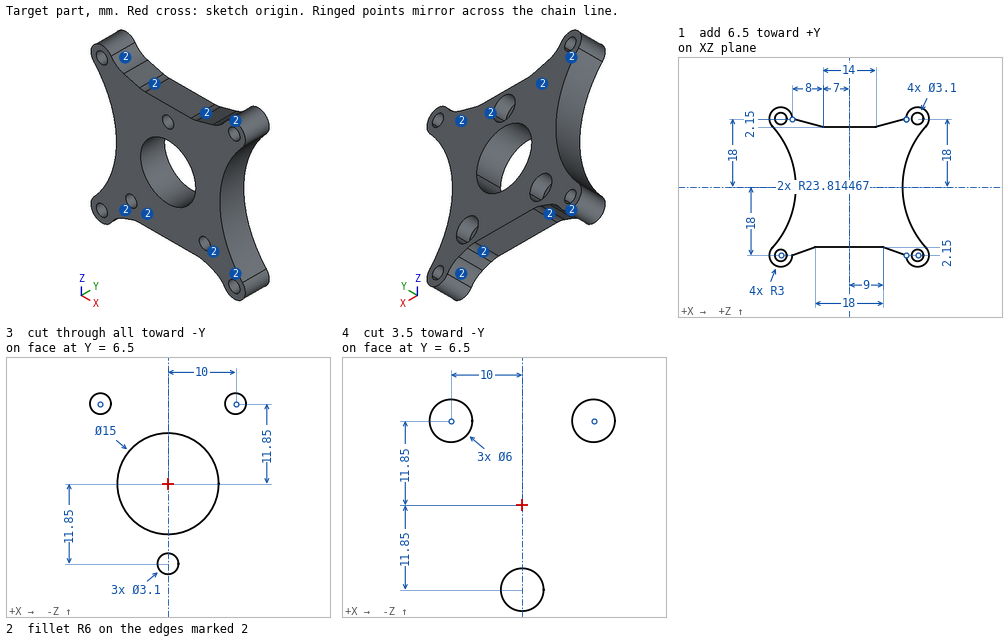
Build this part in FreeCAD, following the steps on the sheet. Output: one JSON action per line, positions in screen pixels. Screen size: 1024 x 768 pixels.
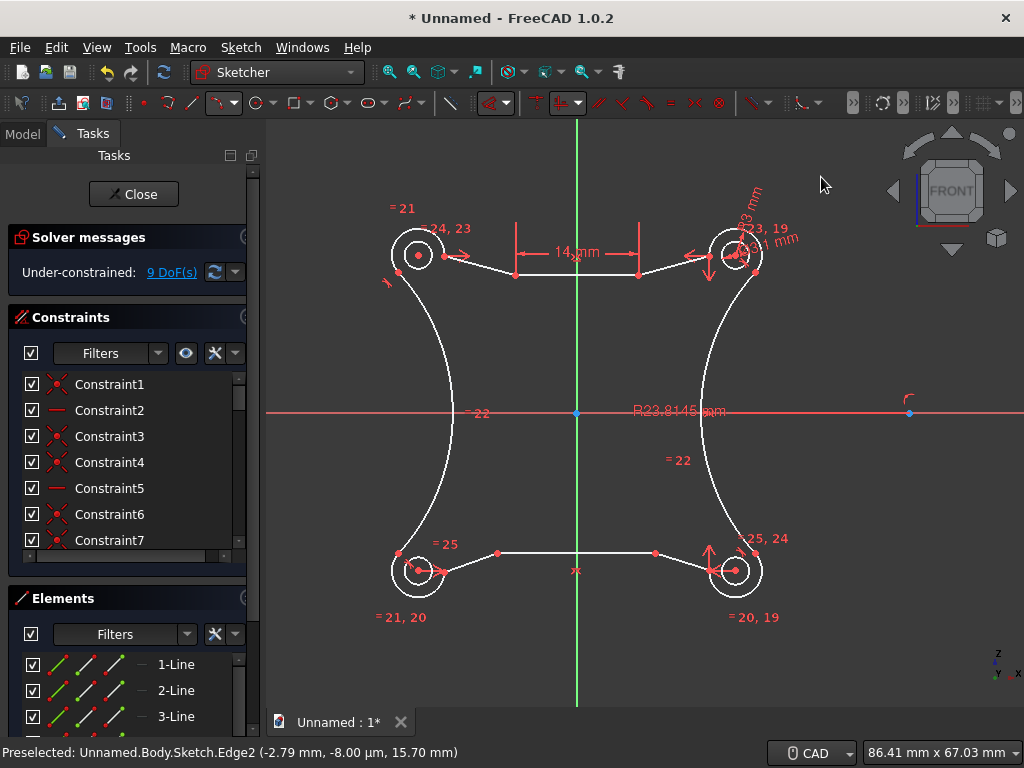
{"action": "left_click", "coordinate": [608, 553]}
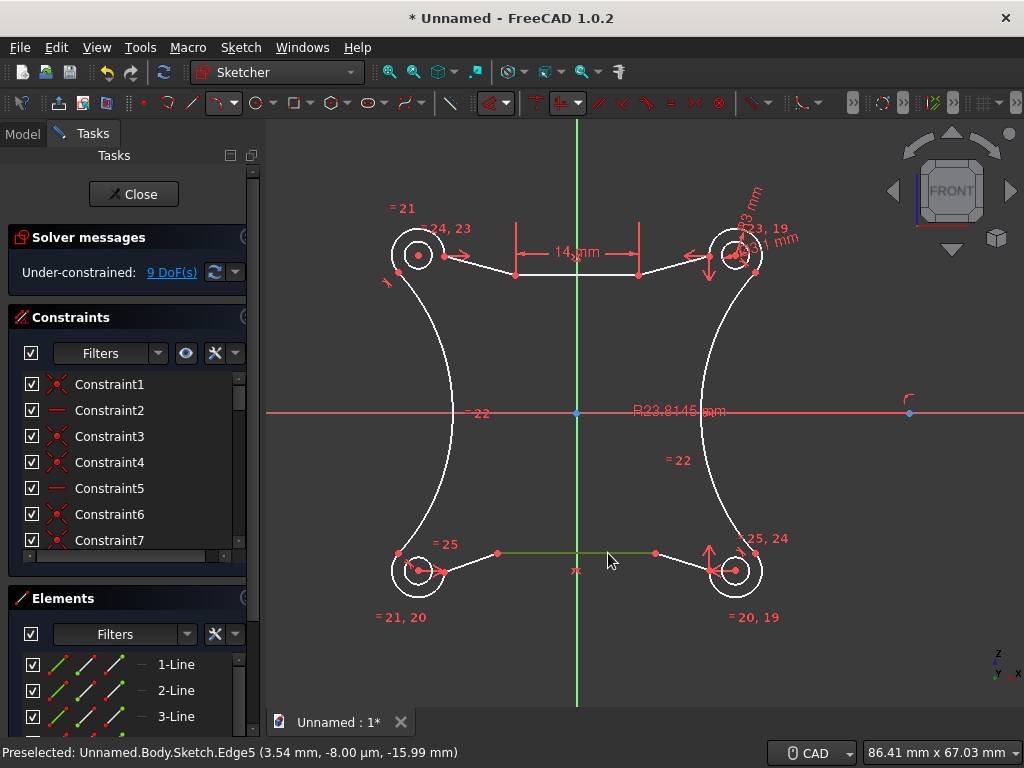
{"action": "left_click", "coordinate": [508, 104]}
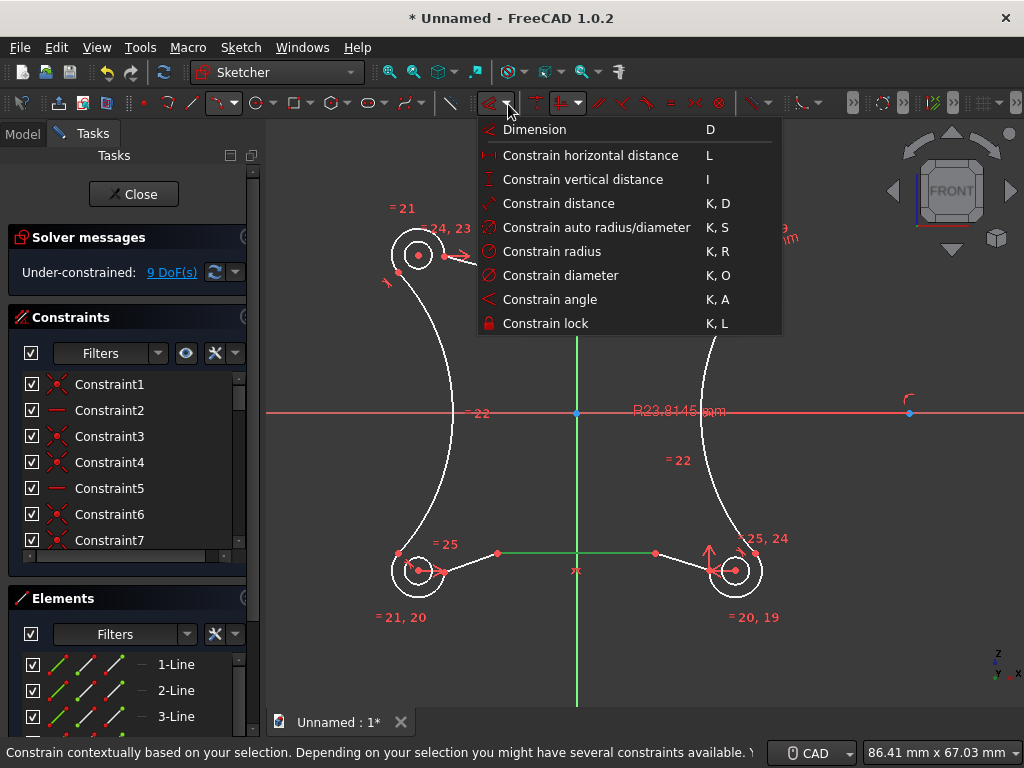
{"action": "left_click", "coordinate": [630, 155]}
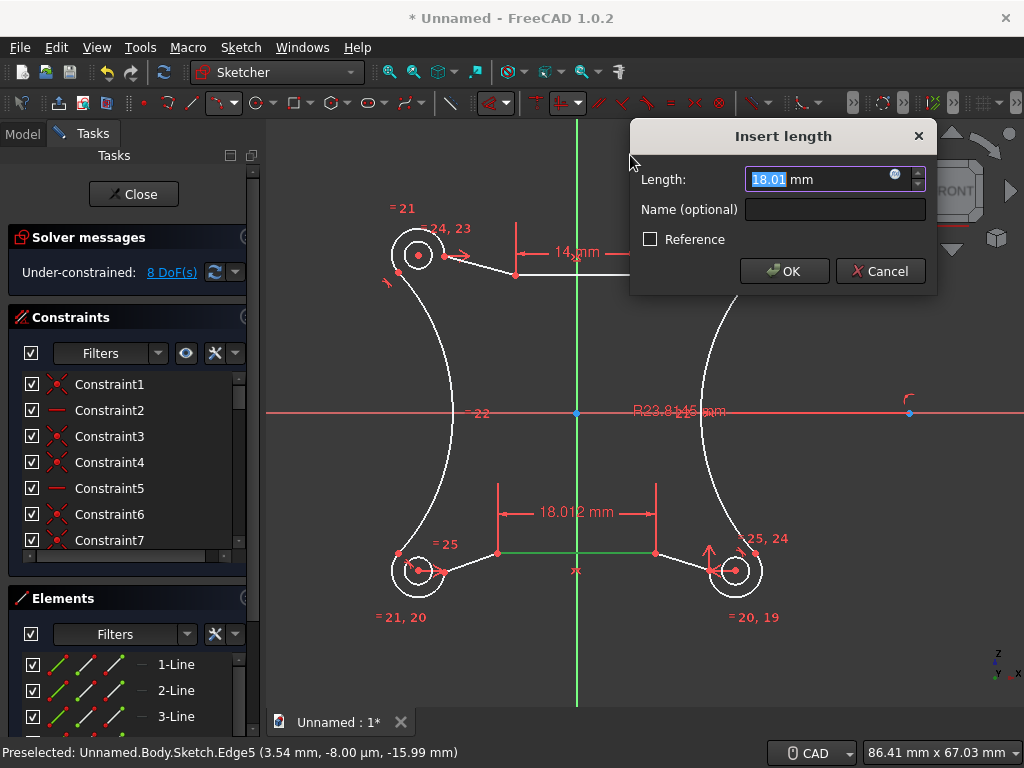
{"action": "type", "text": "18"}
{"action": "key", "text": "Return"}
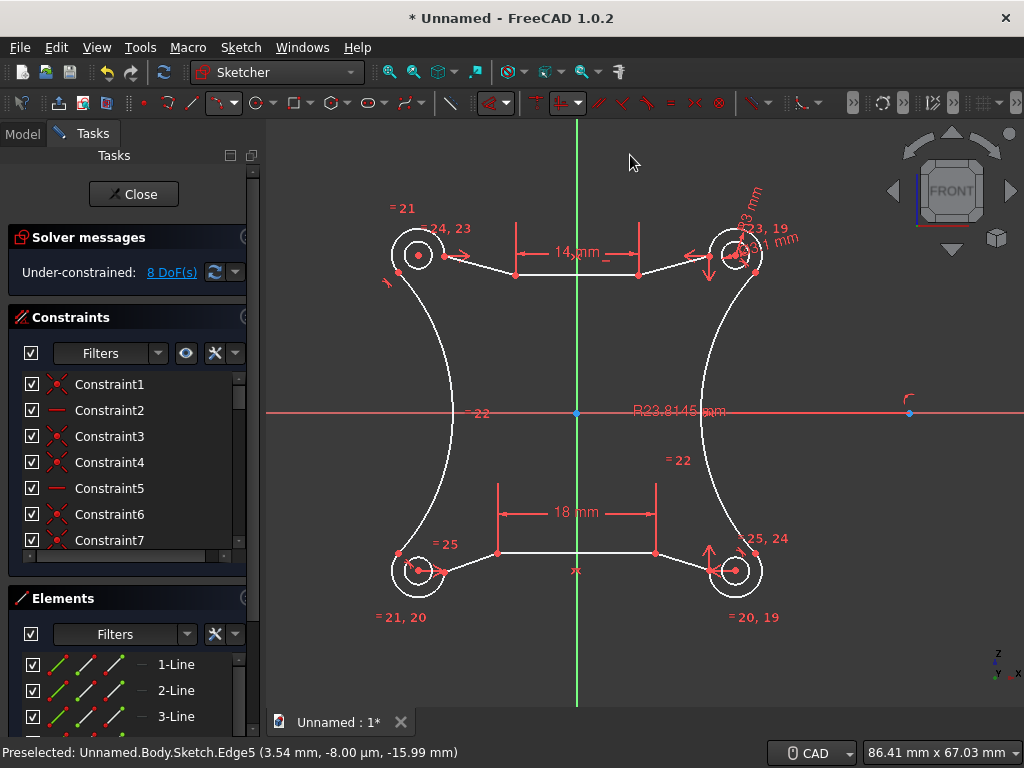
{"action": "left_click", "coordinate": [516, 275]}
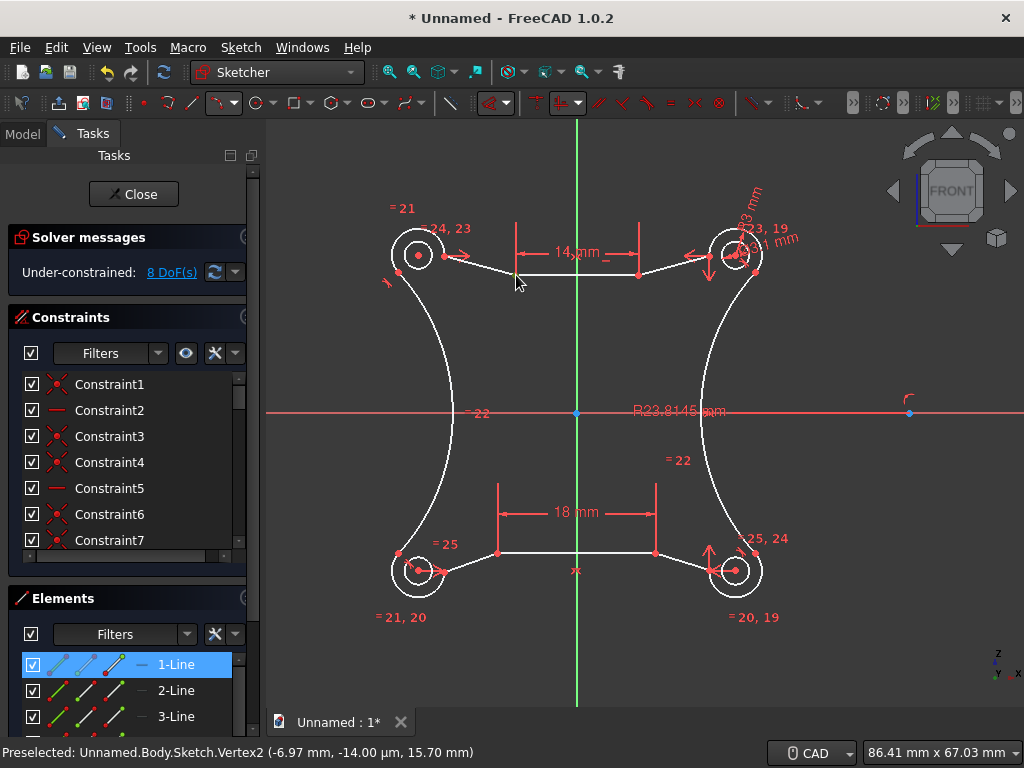
{"action": "key", "text": "l"}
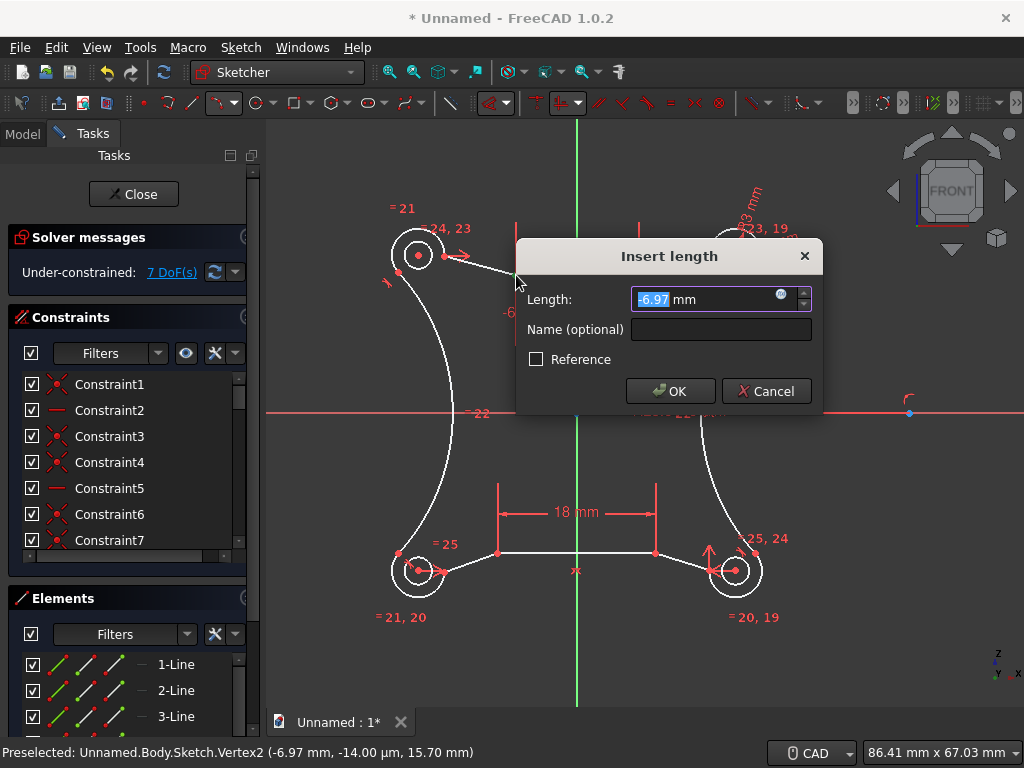
{"action": "type", "text": "-7"}
{"action": "key", "text": "Return"}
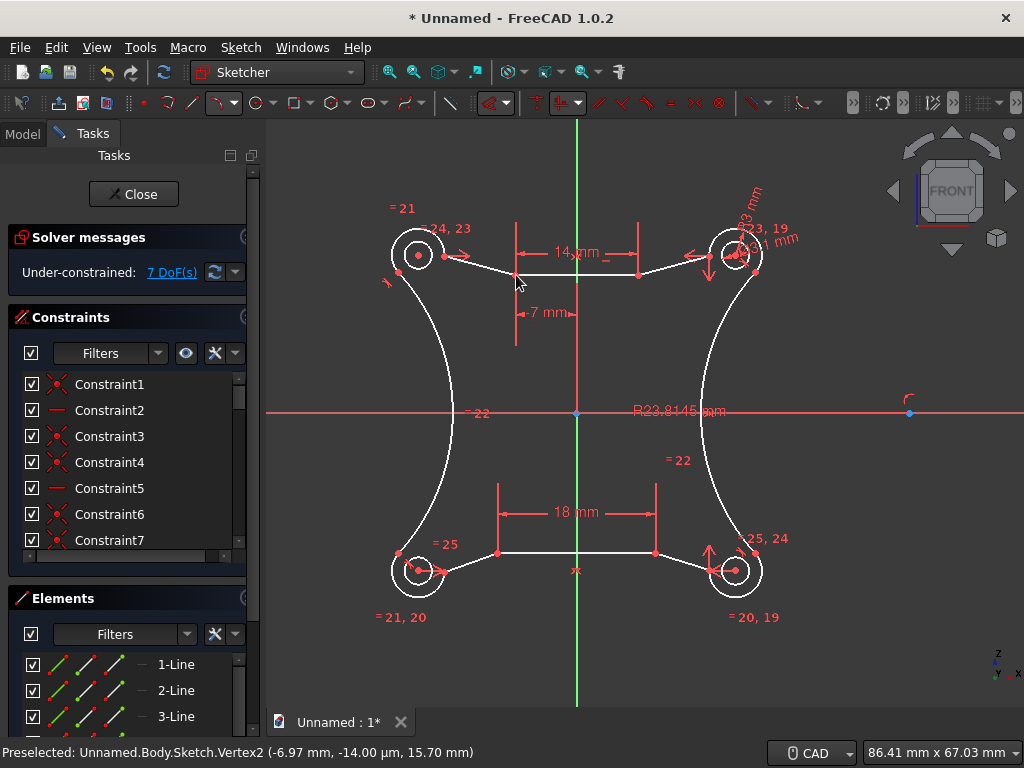
{"action": "left_click", "coordinate": [656, 553]}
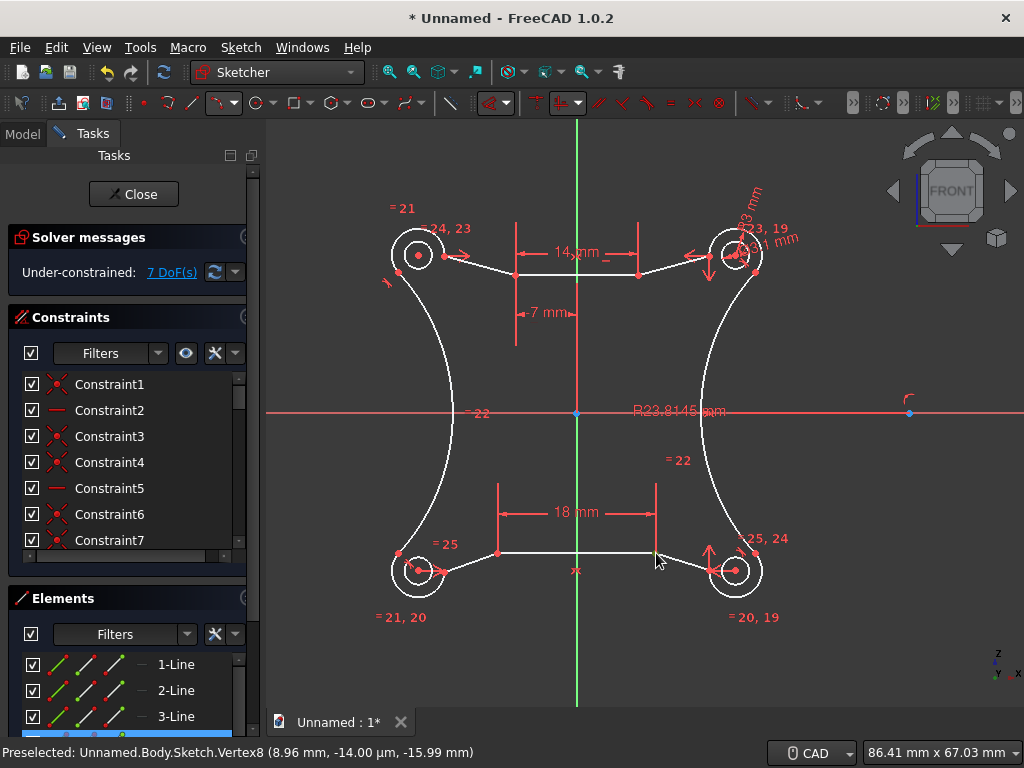
{"action": "key", "text": "l"}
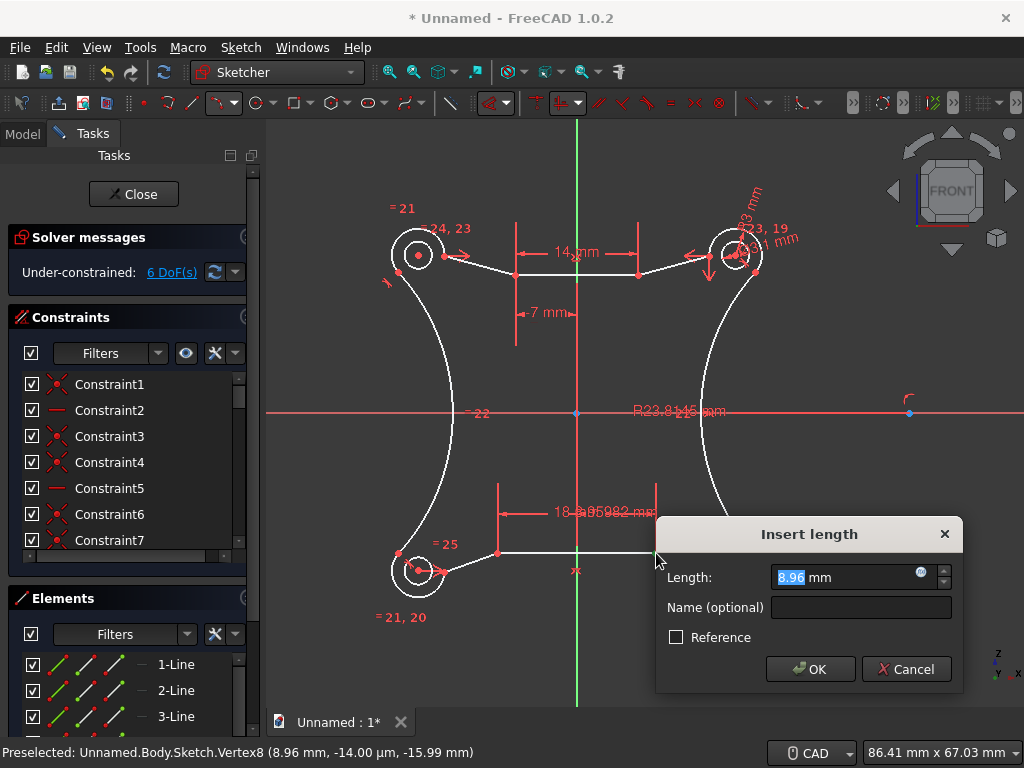
{"action": "type", "text": "9"}
{"action": "key", "text": "Return"}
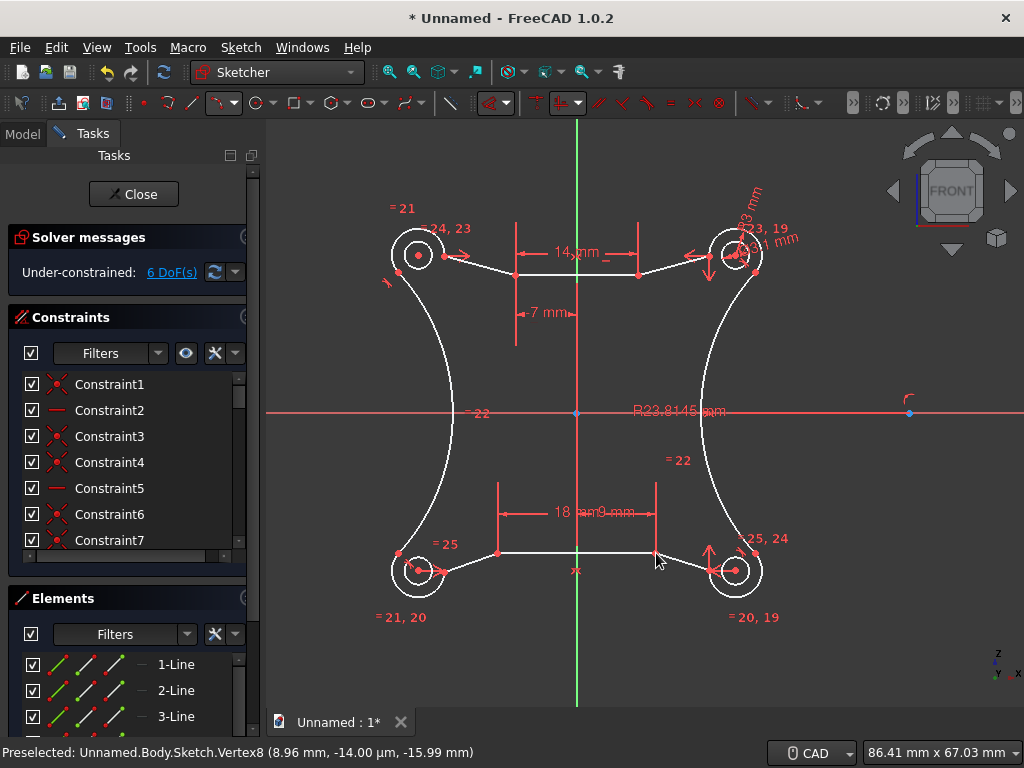
{"action": "left_click", "coordinate": [466, 262]}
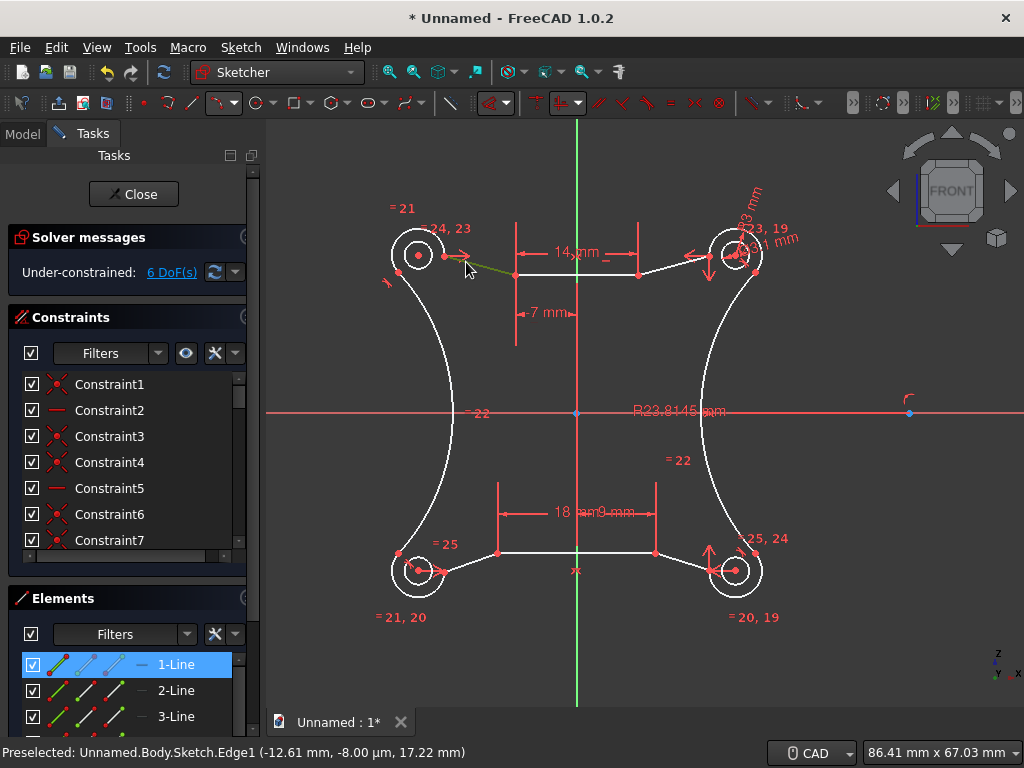
{"action": "left_click", "coordinate": [508, 104]}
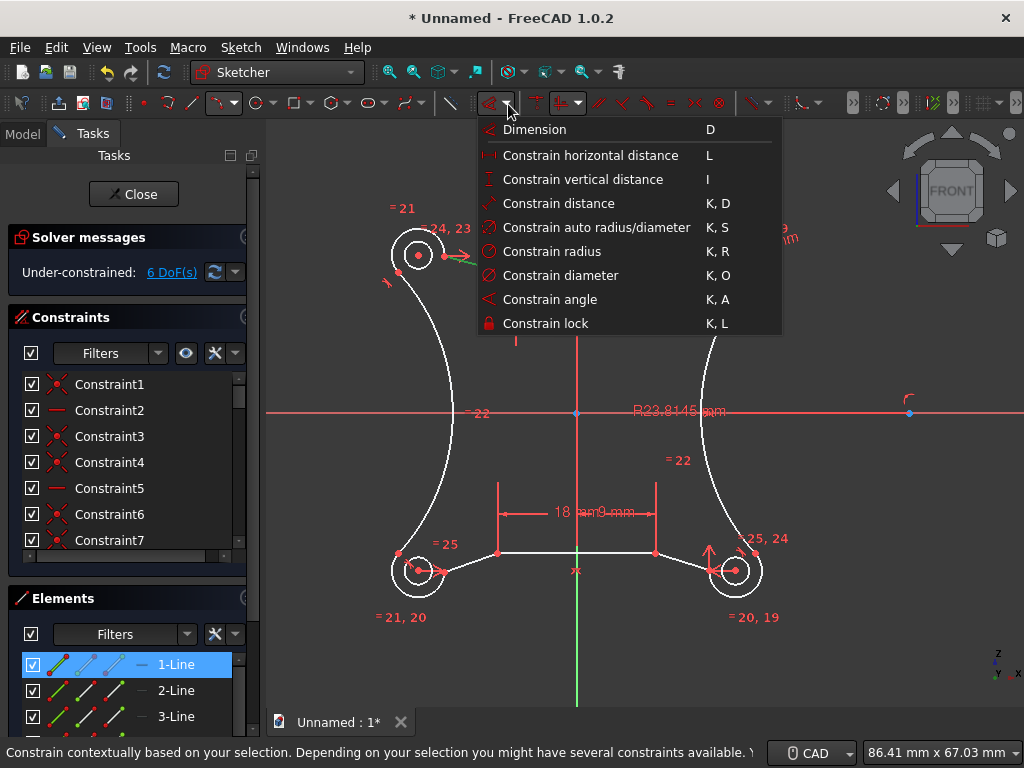
{"action": "left_click", "coordinate": [630, 155]}